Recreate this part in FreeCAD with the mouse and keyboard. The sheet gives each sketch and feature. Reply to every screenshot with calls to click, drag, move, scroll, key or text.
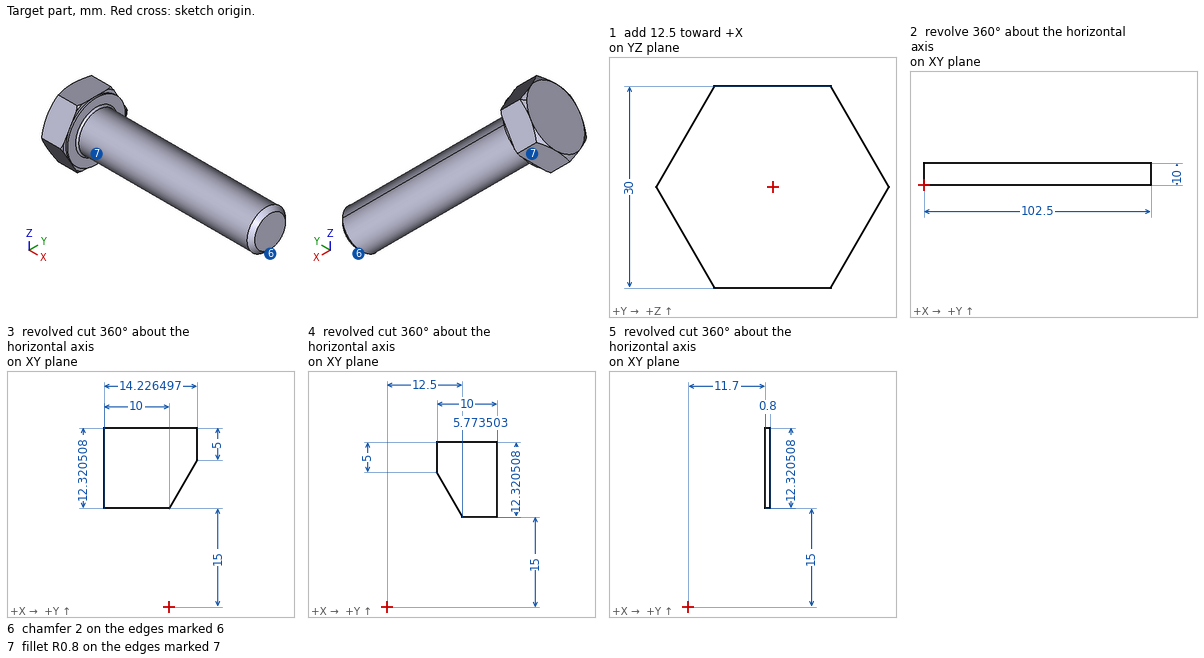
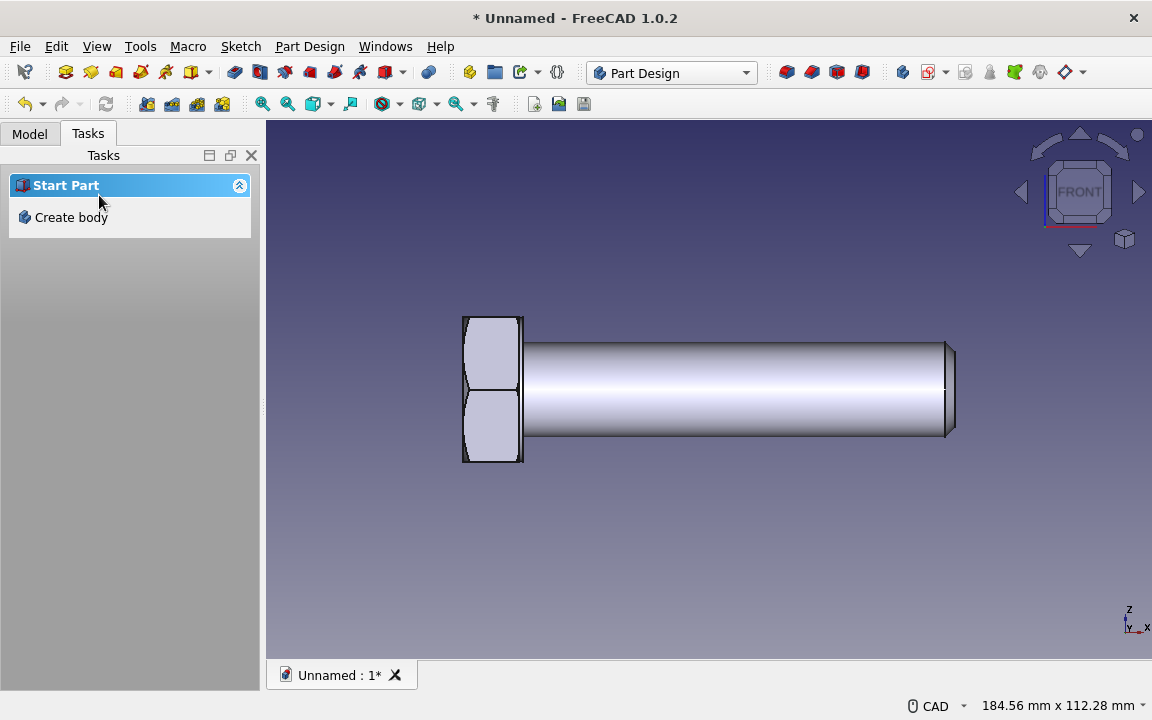
key(3)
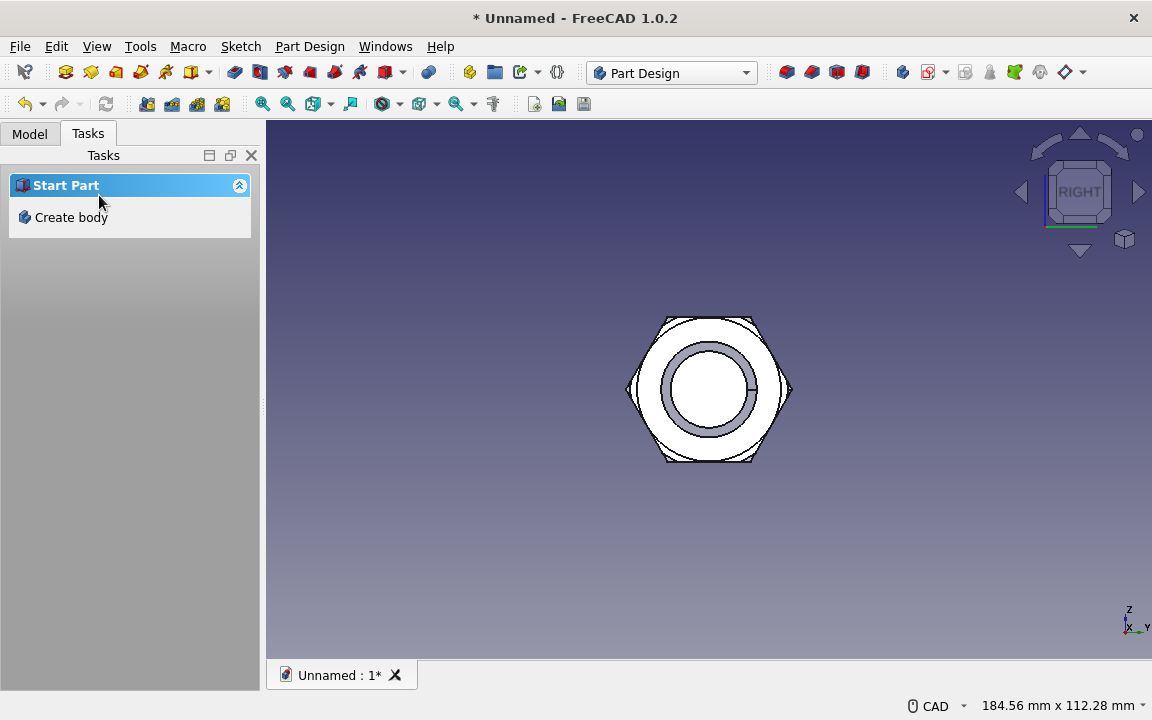
click(263, 104)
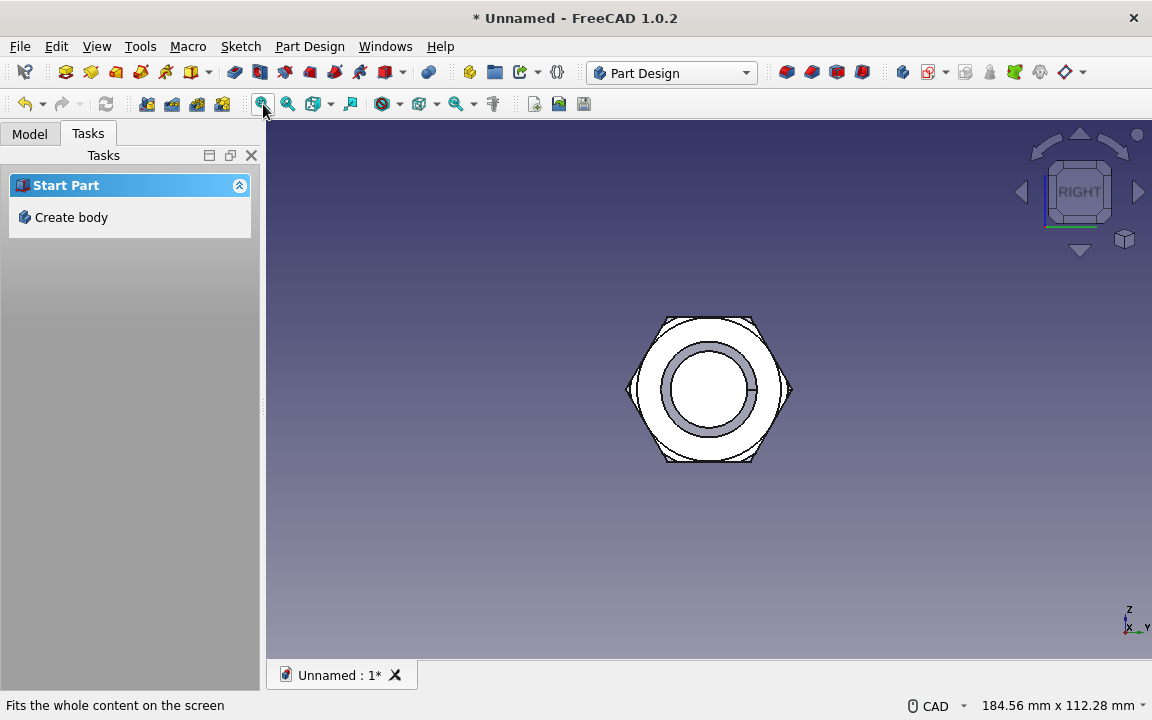
key(5)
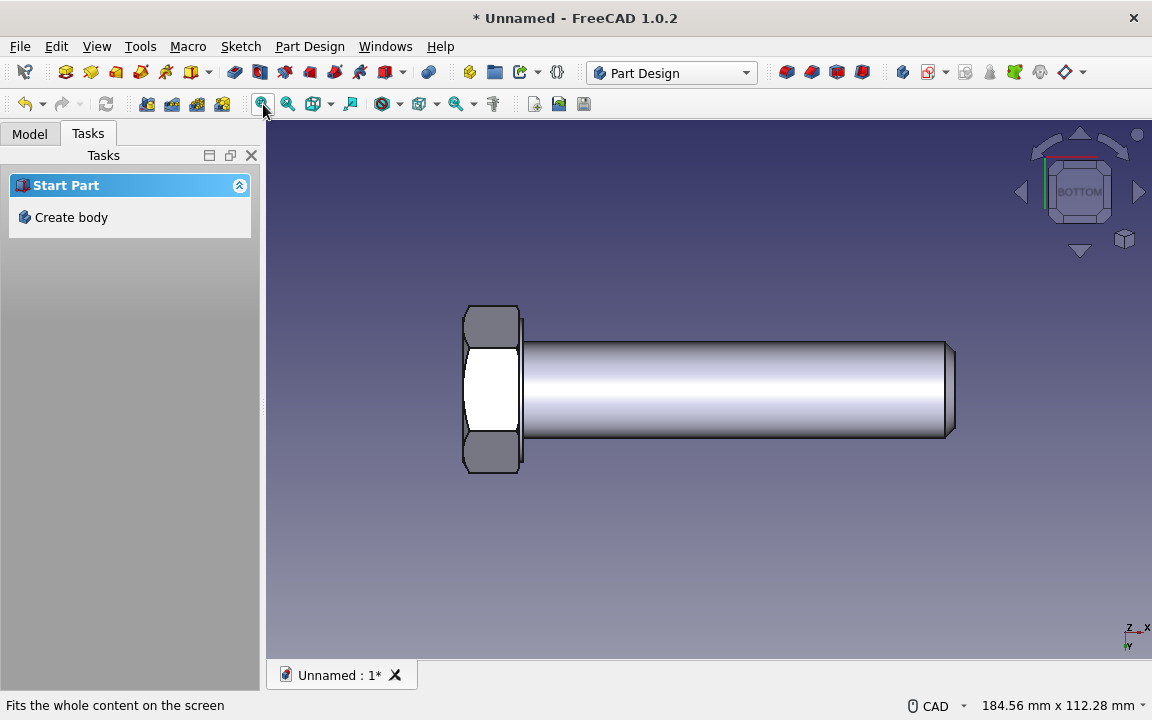
key(4)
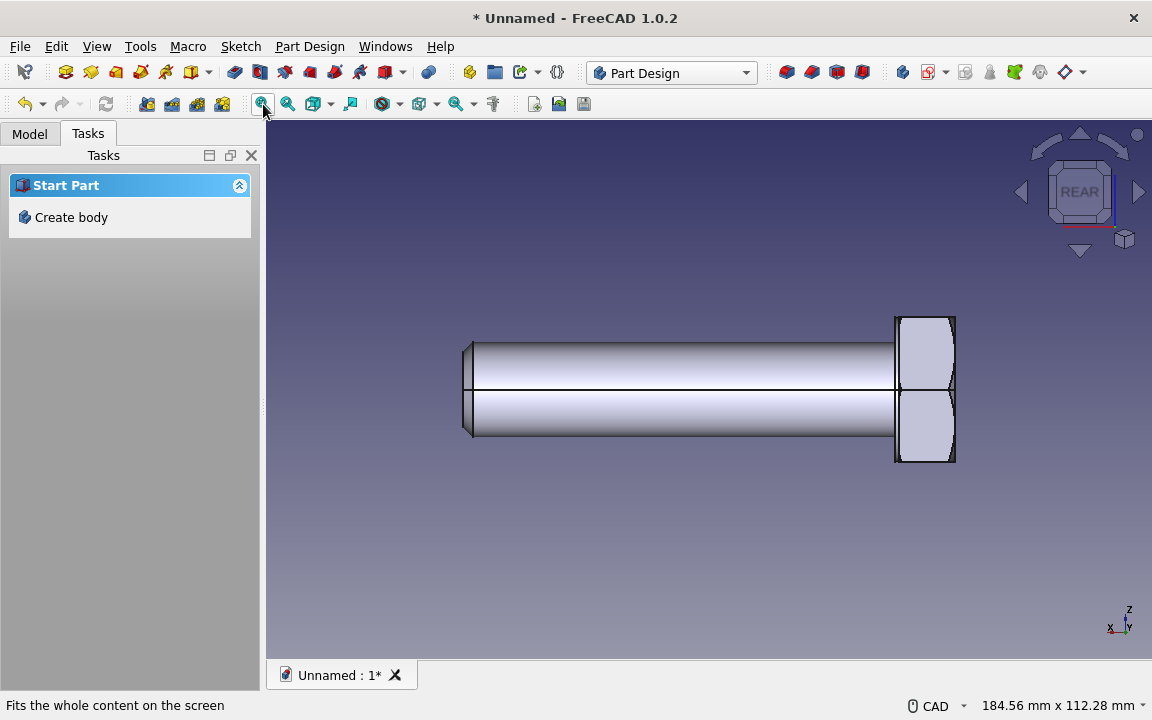
key(6)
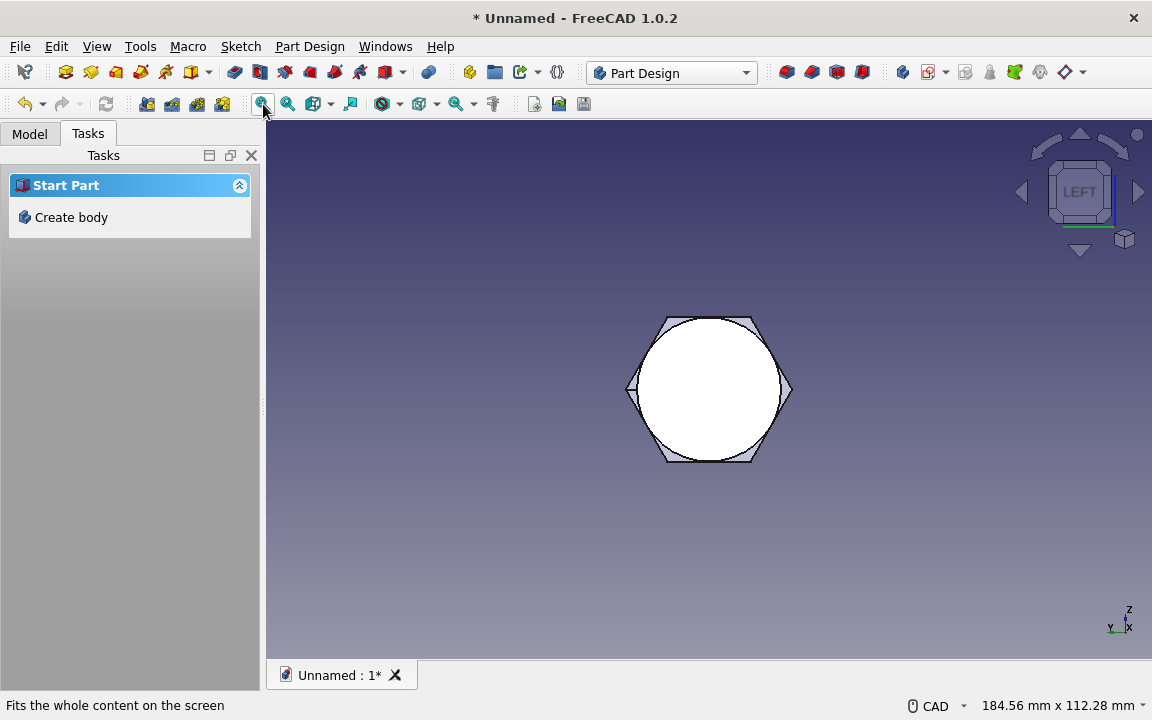
key(v)
key(f)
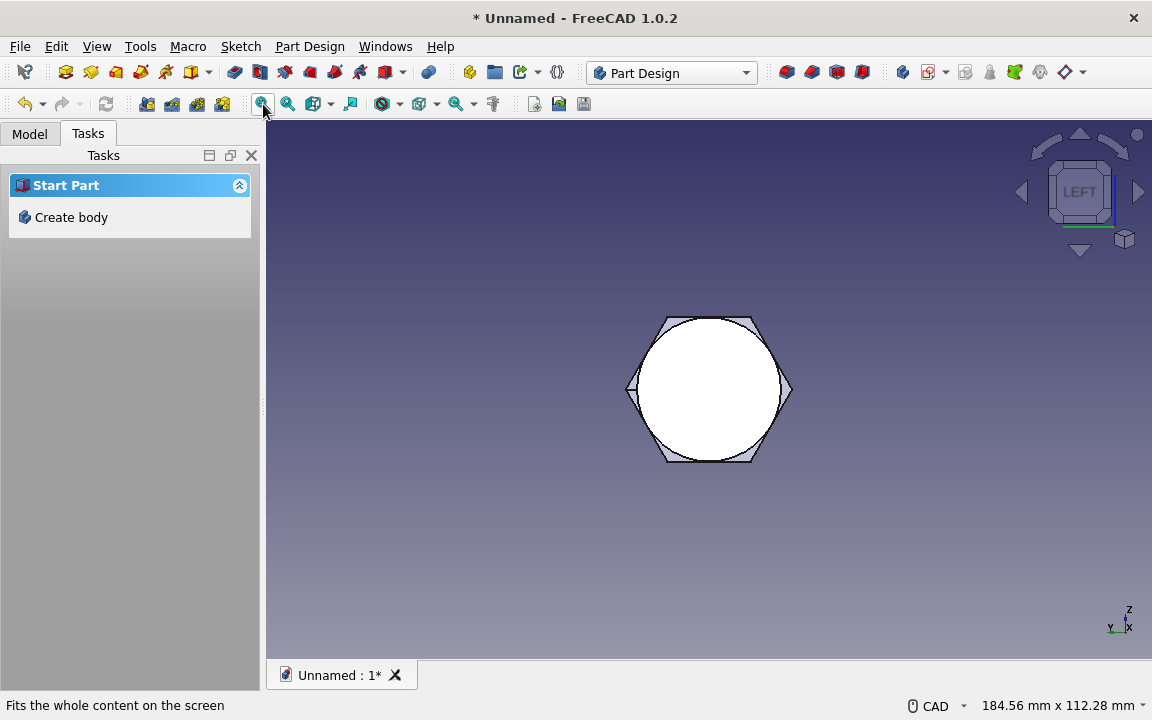
key(v)
key(3)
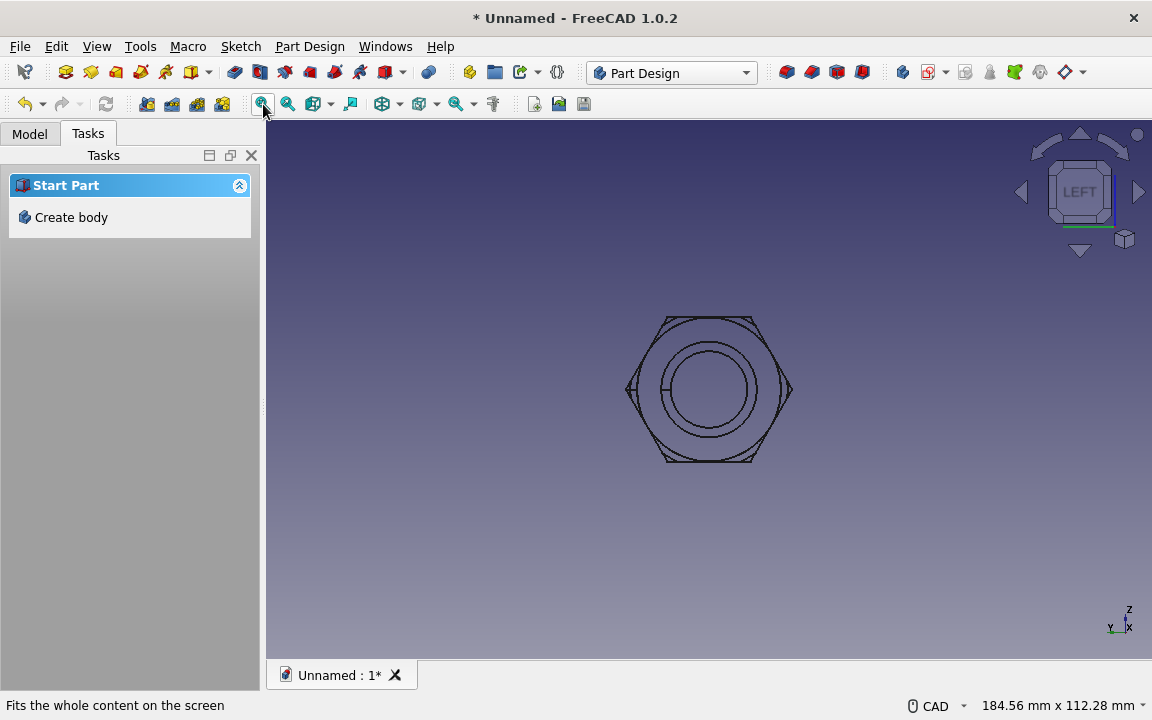
key(0)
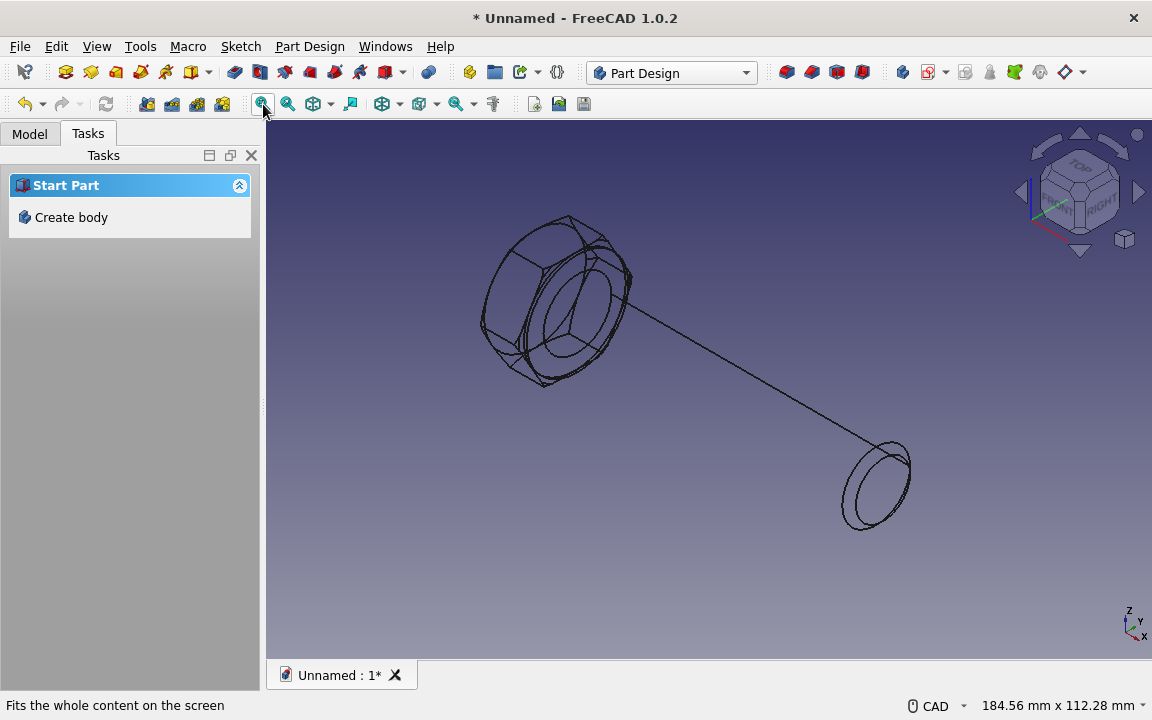
click(544, 332)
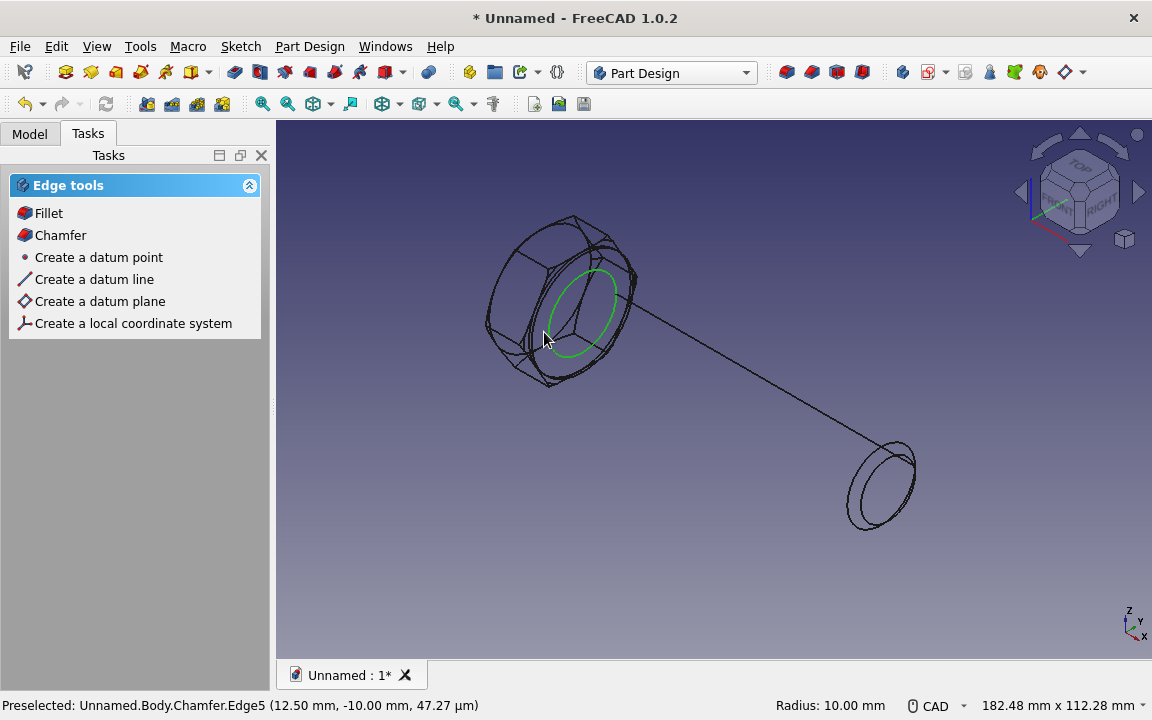
key(v)
key(1)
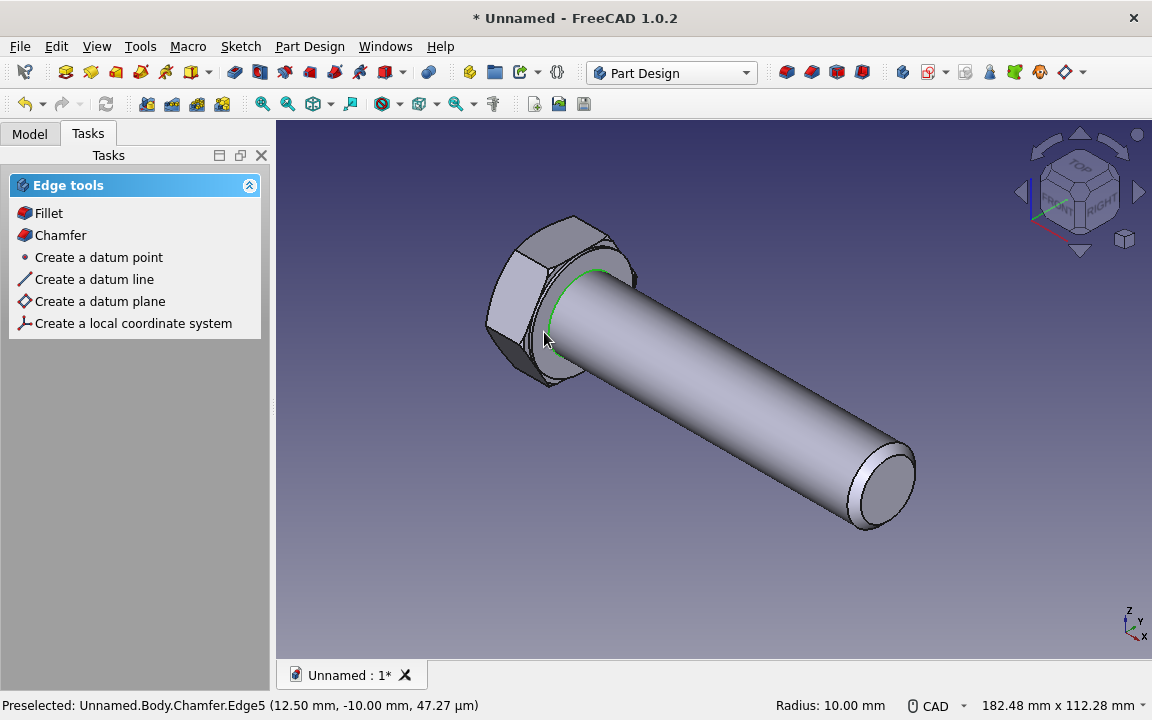
click(787, 72)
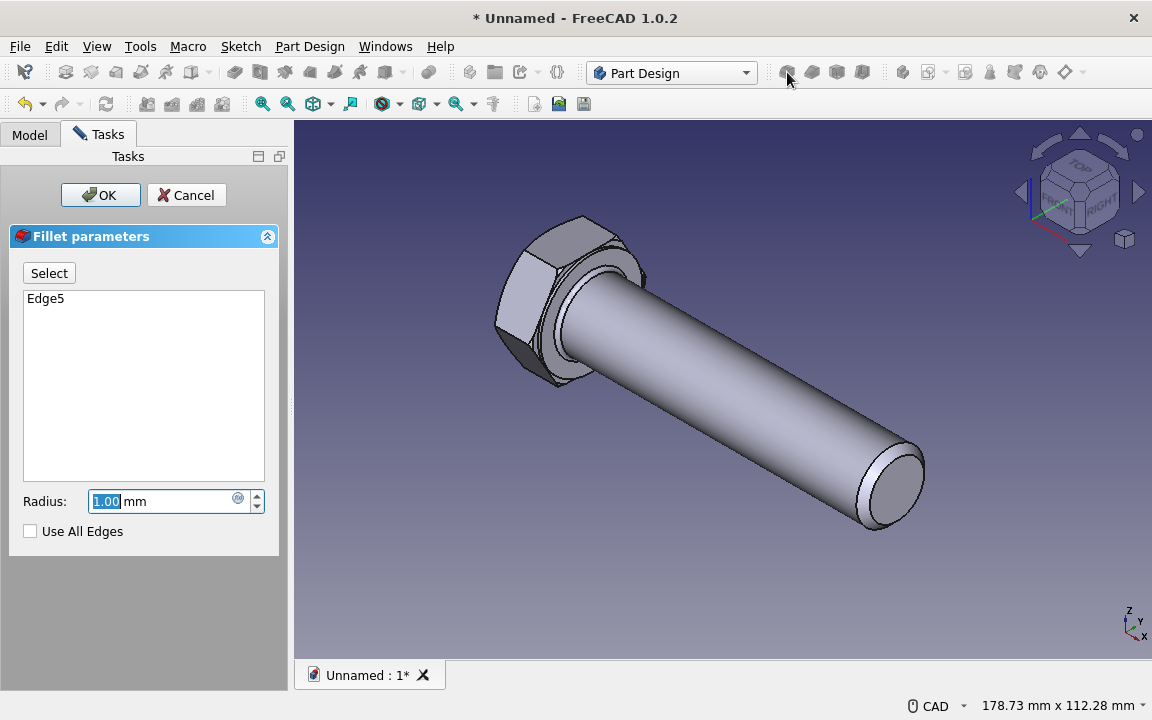
text(0.8)
key(Tab)